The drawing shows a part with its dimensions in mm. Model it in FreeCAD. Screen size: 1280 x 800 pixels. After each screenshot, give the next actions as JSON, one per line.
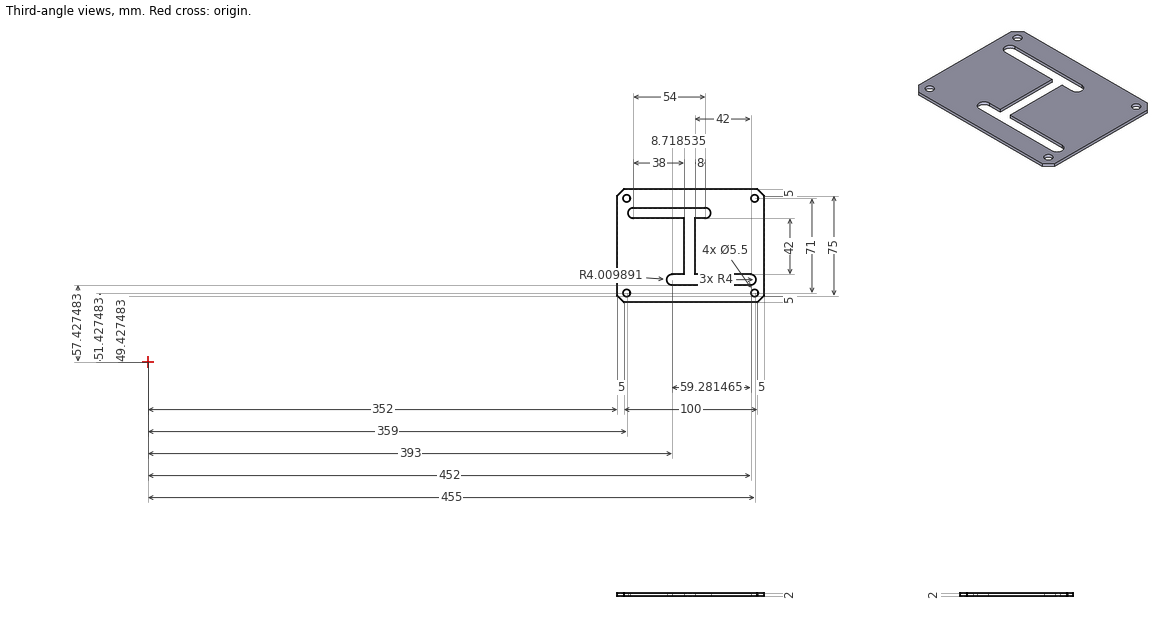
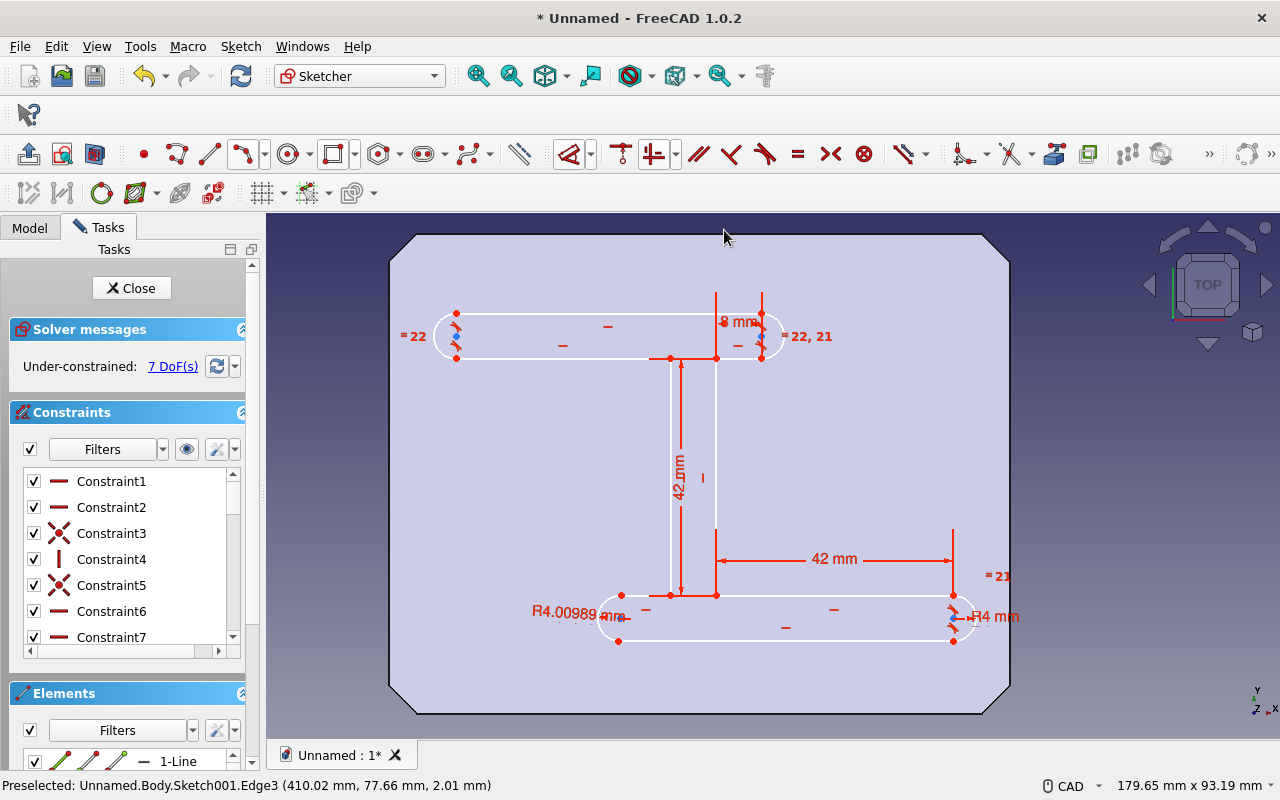
{"action": "left_click", "coordinate": [670, 314]}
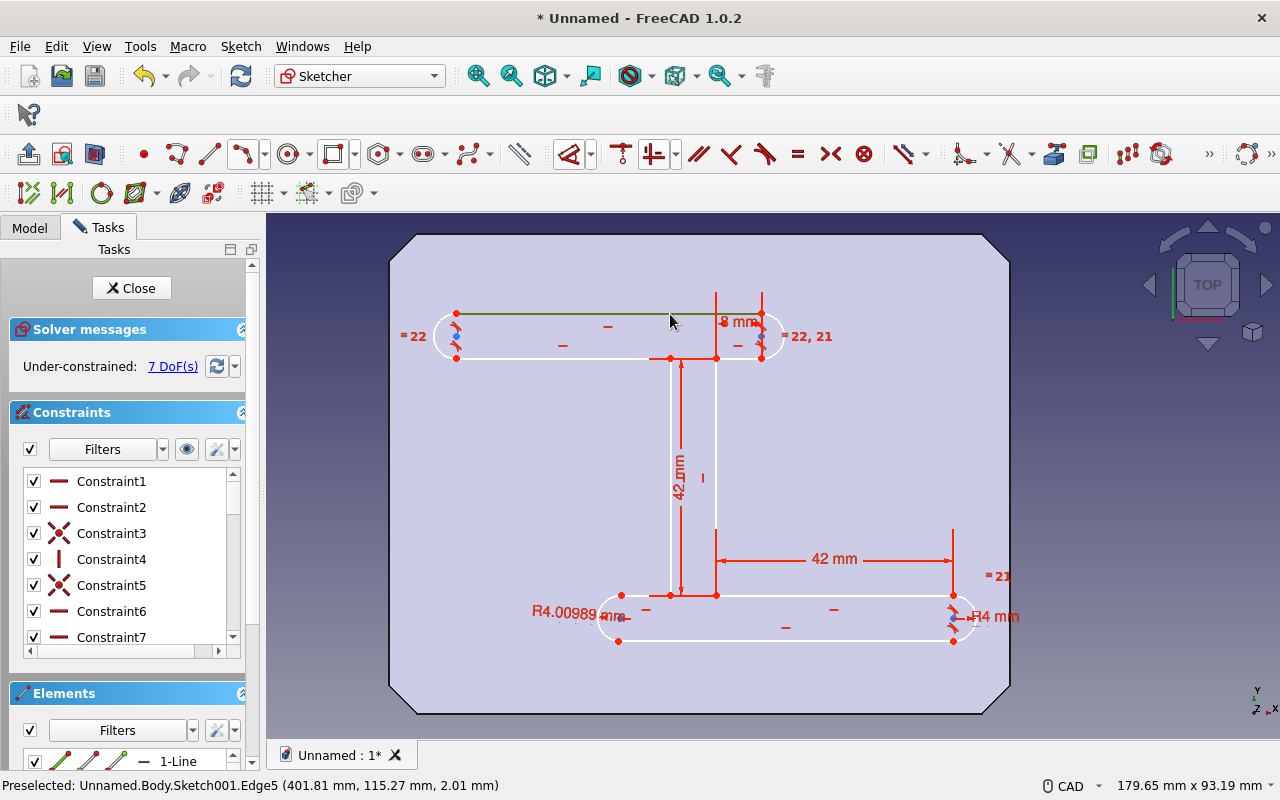
{"action": "left_click", "coordinate": [590, 154]}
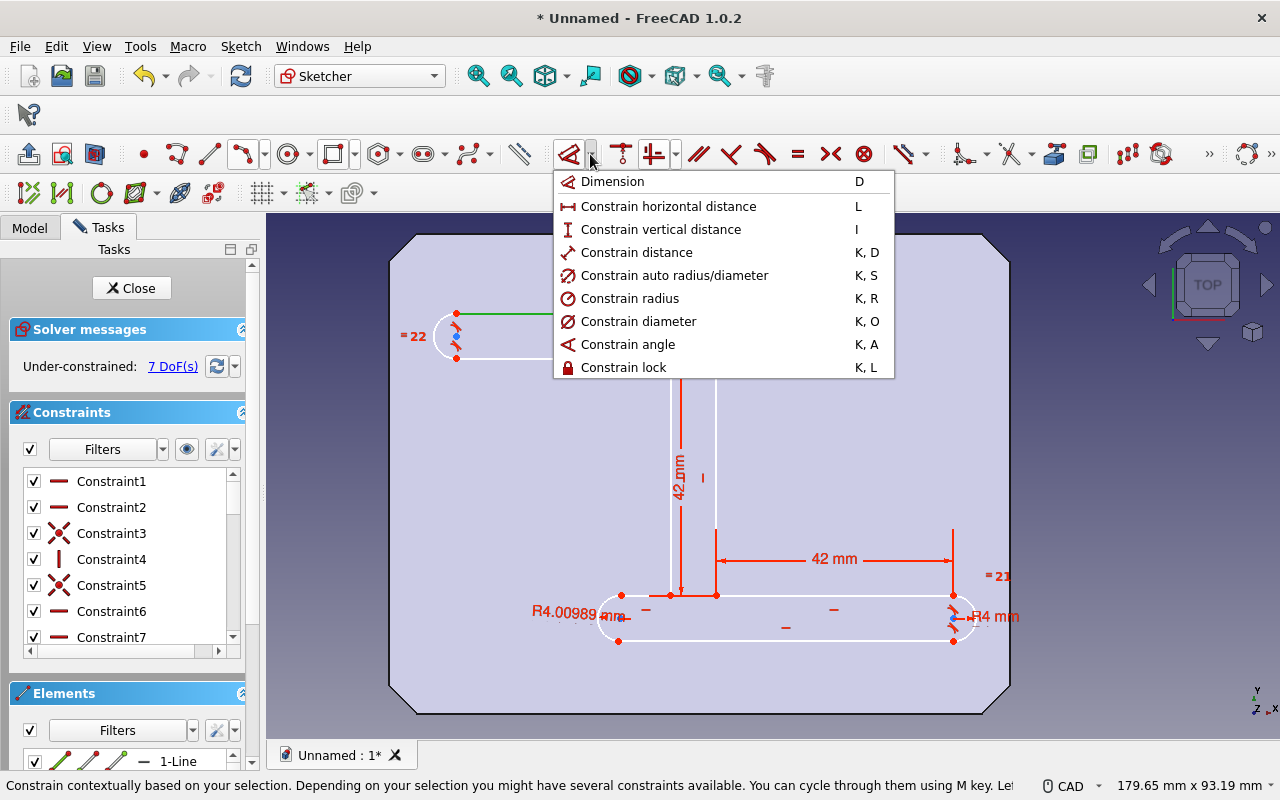
{"action": "left_click", "coordinate": [724, 206]}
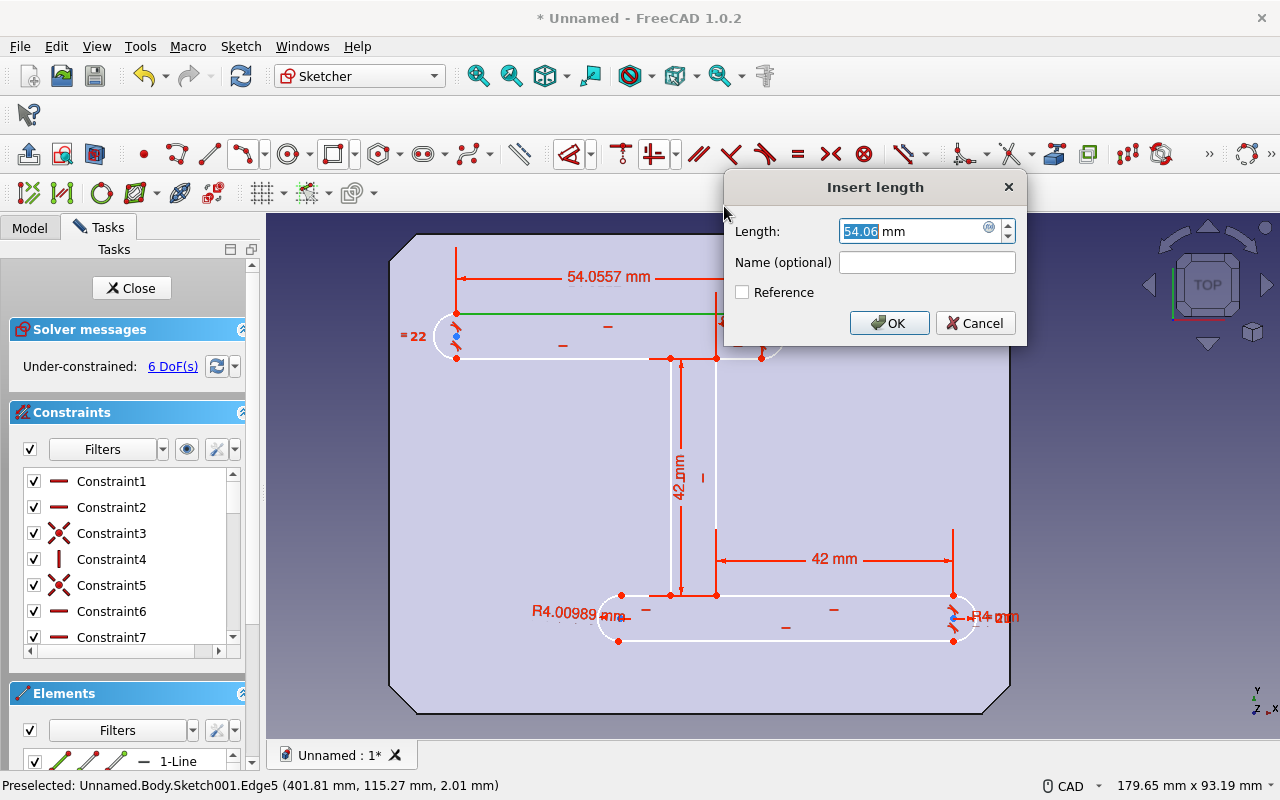
{"action": "type", "text": "54"}
{"action": "key", "text": "Return"}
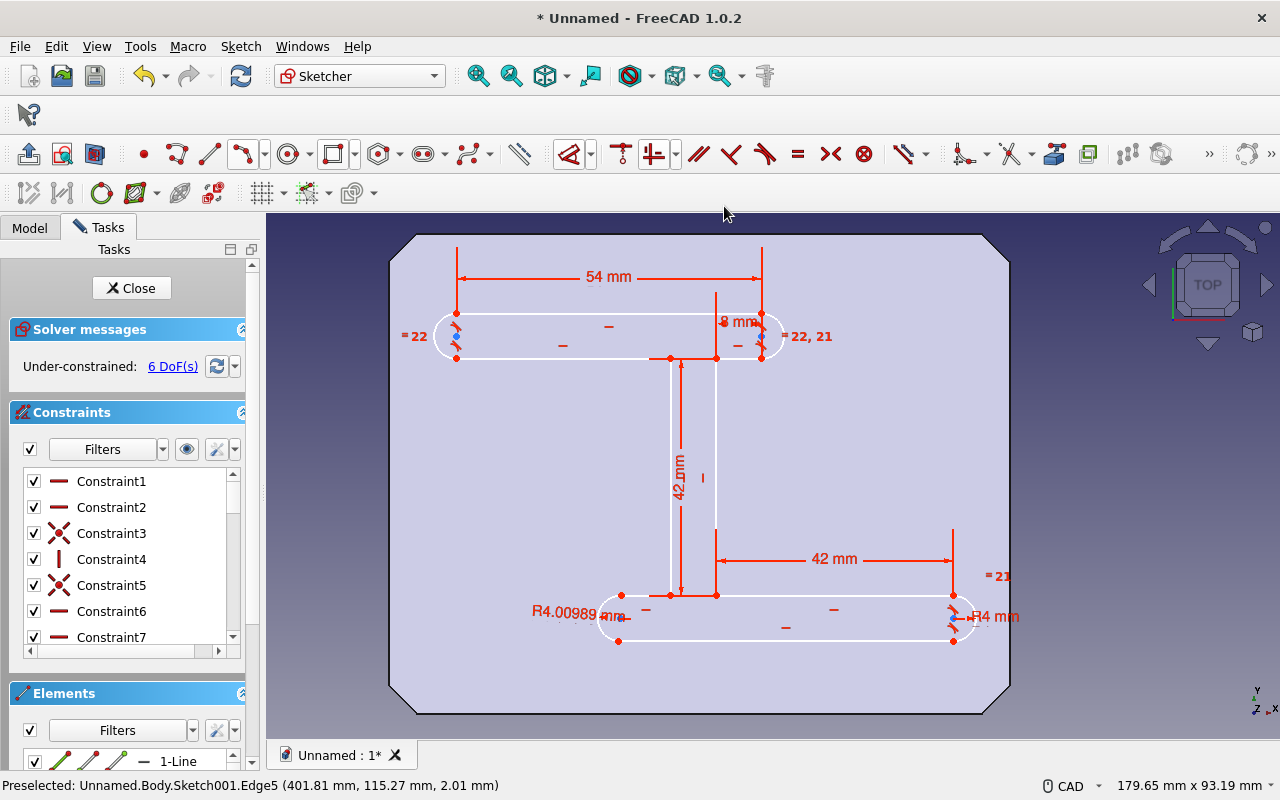
{"action": "left_click", "coordinate": [521, 359]}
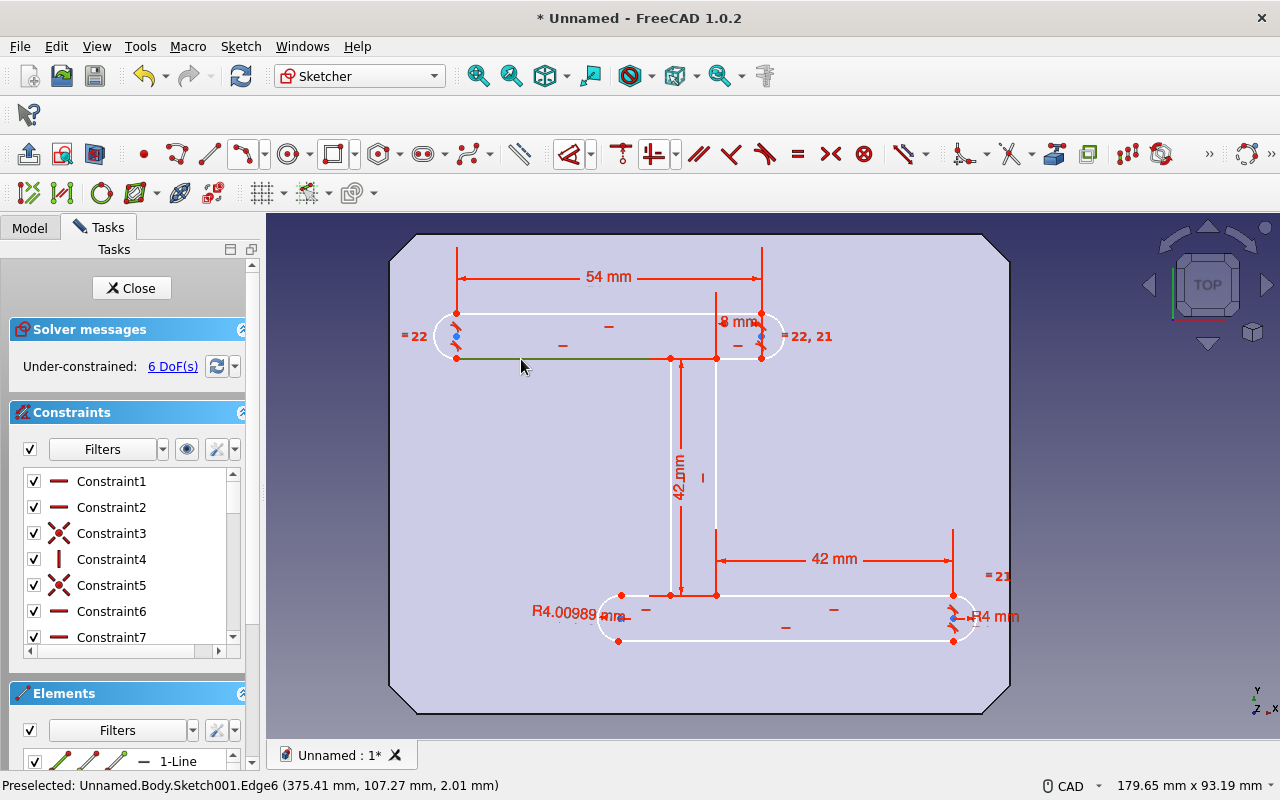
{"action": "key", "text": "l"}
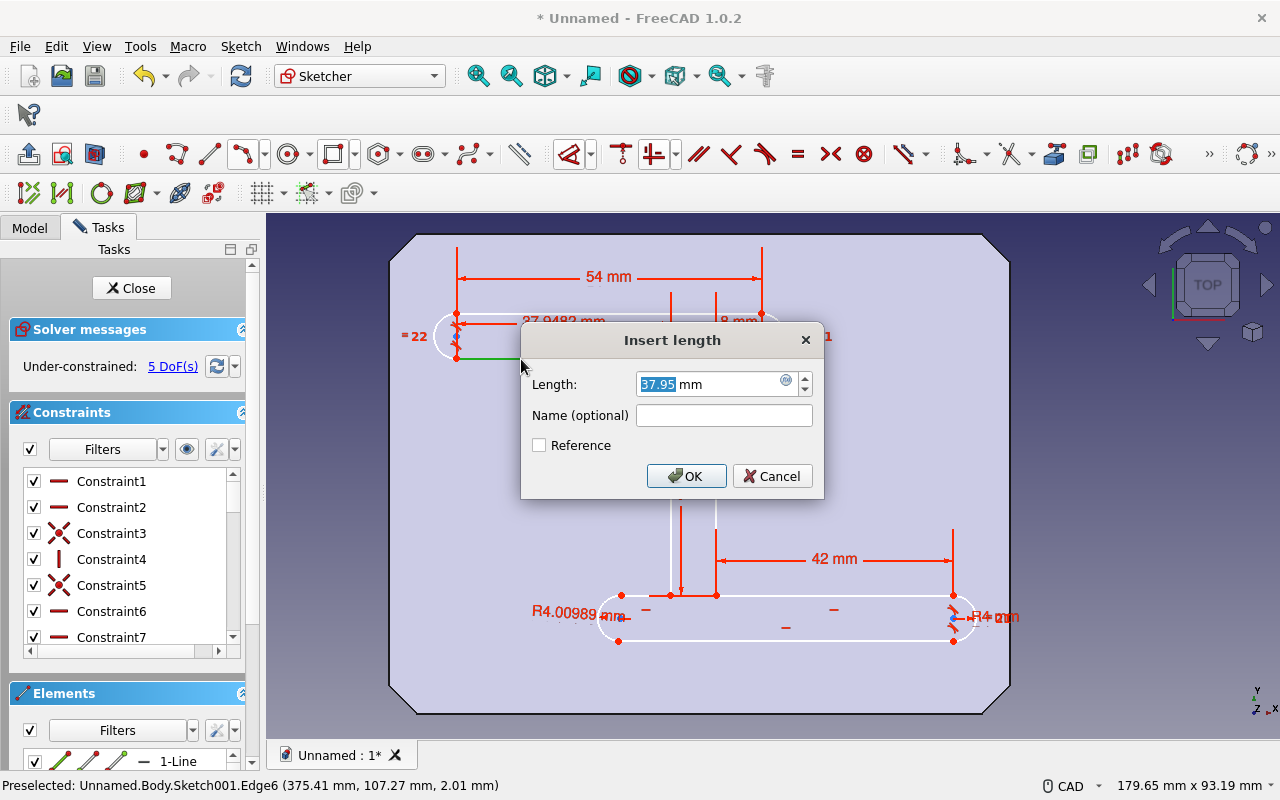
{"action": "type", "text": "38"}
{"action": "key", "text": "Return"}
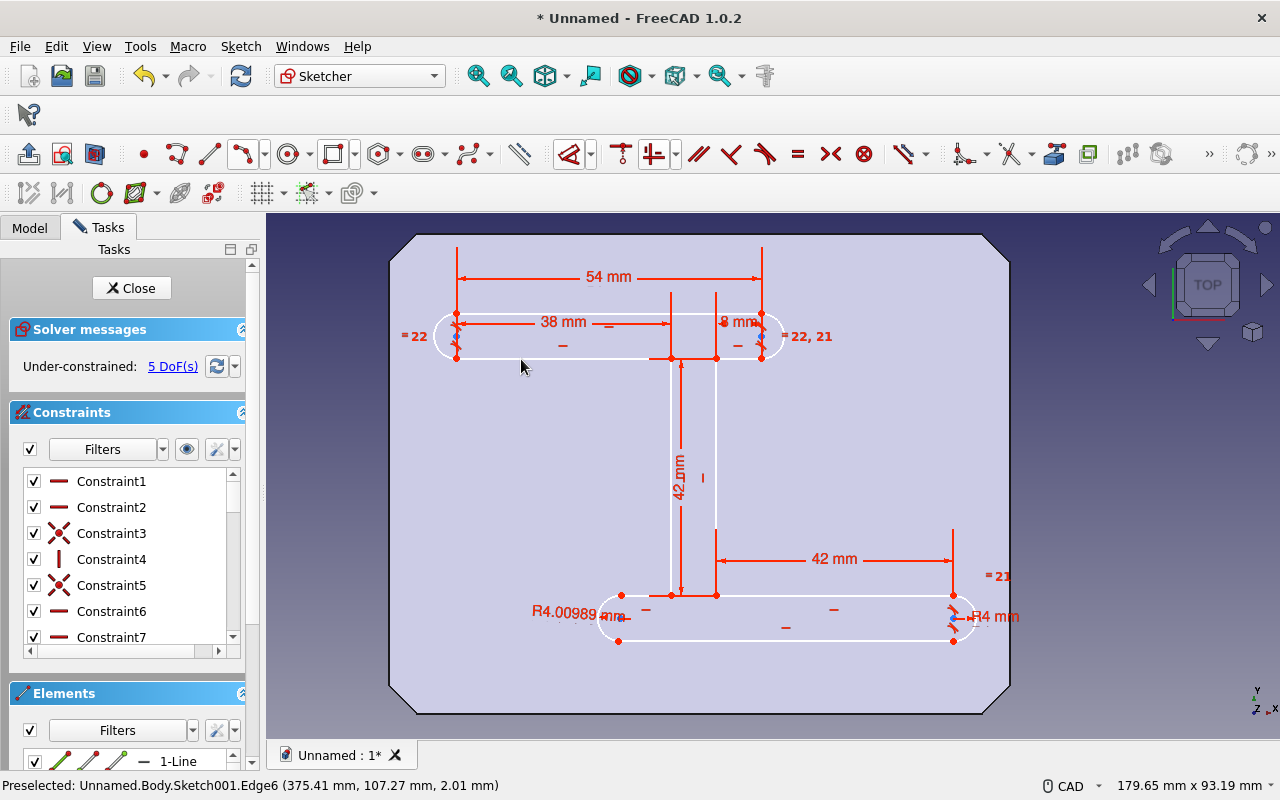
{"action": "left_click", "coordinate": [953, 641]}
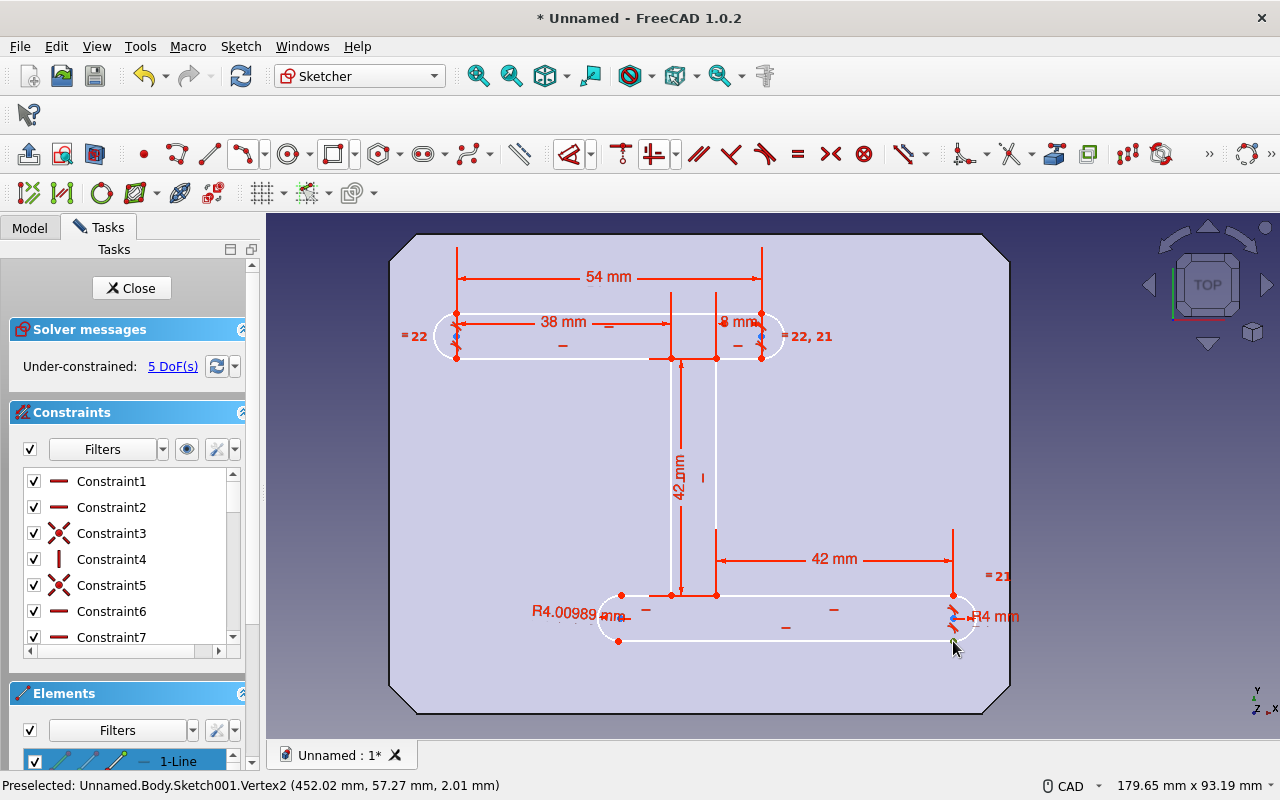
{"action": "key", "text": "l"}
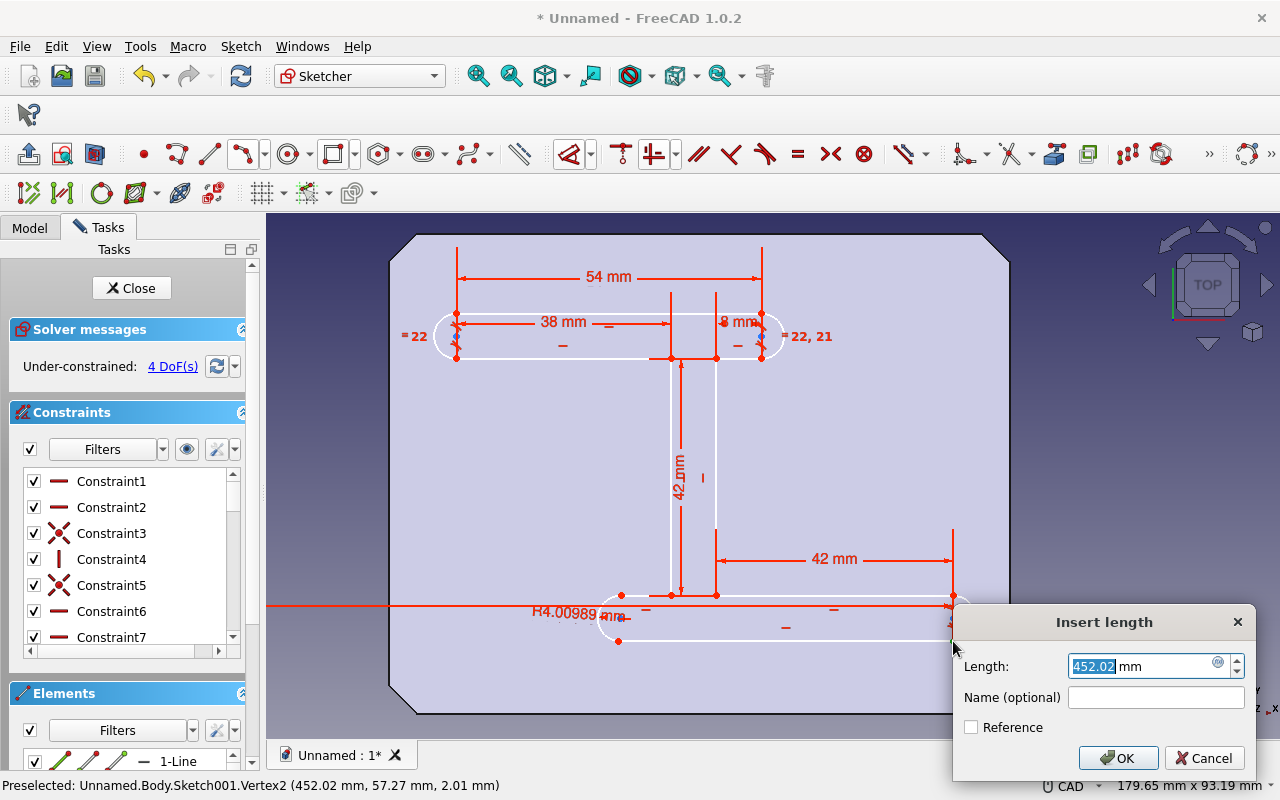
{"action": "type", "text": "452"}
{"action": "key", "text": "Return"}